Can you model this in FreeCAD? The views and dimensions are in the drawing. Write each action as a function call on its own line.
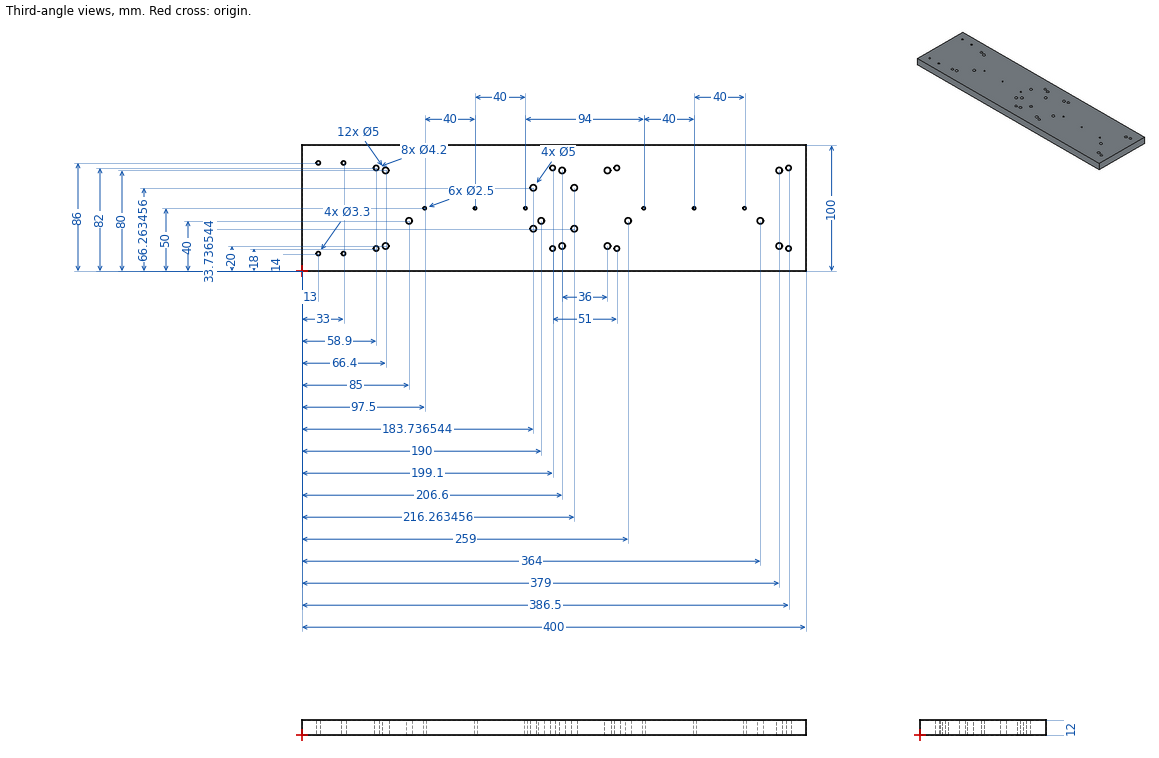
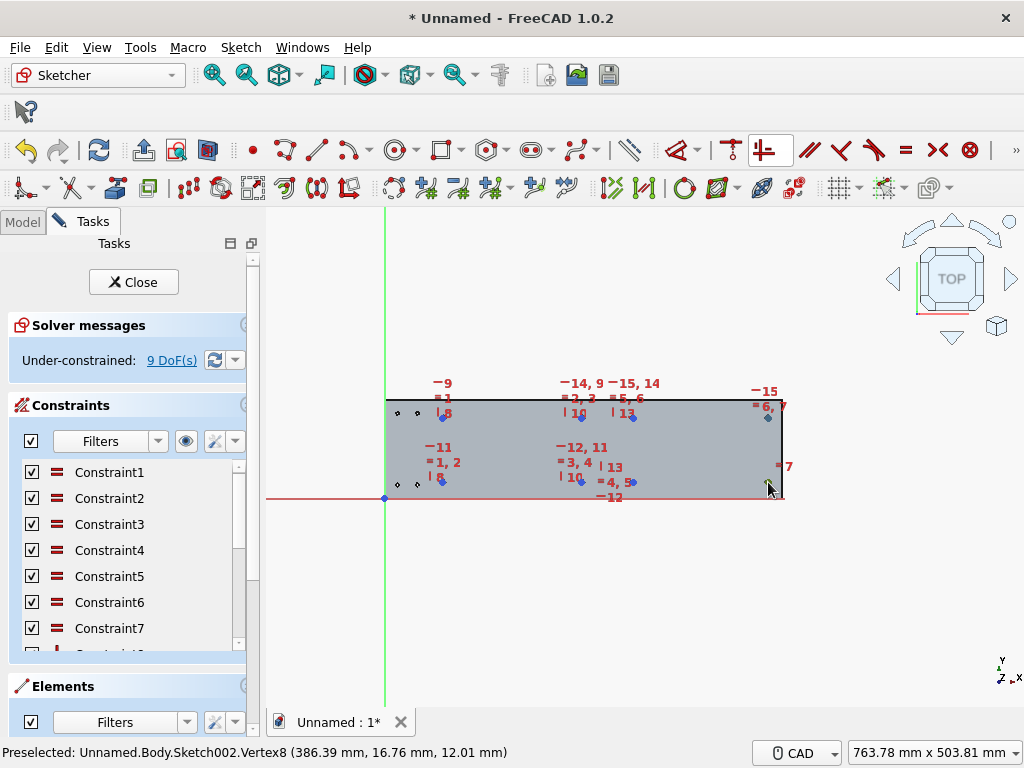
click(788, 150)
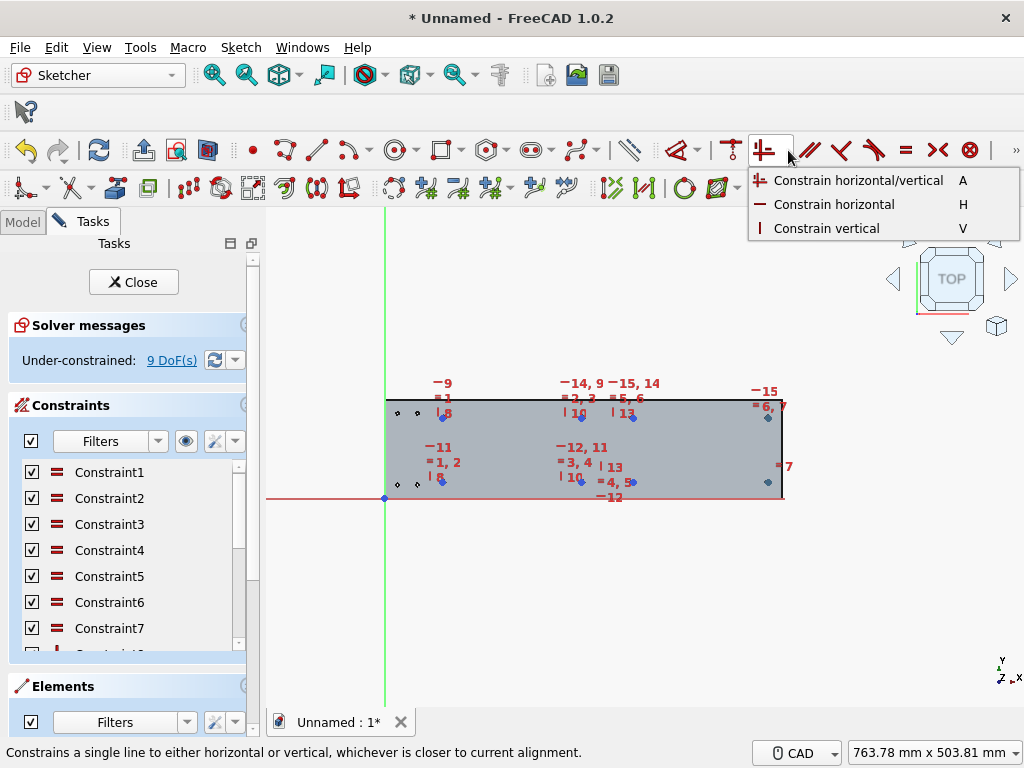
click(884, 228)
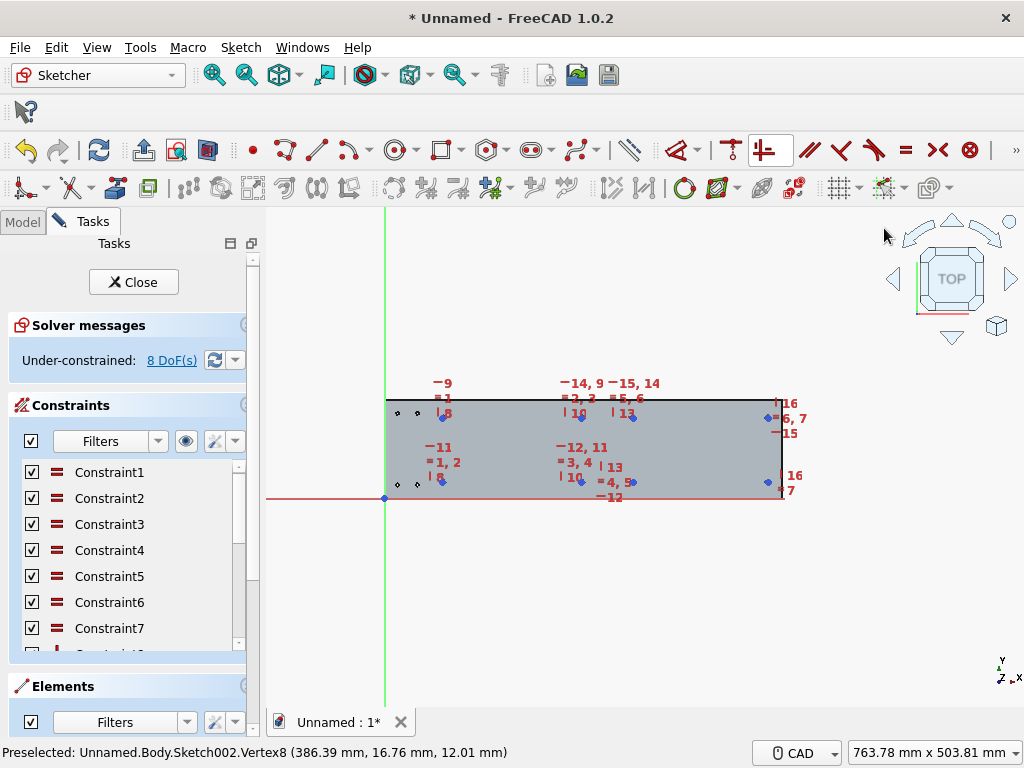
click(633, 482)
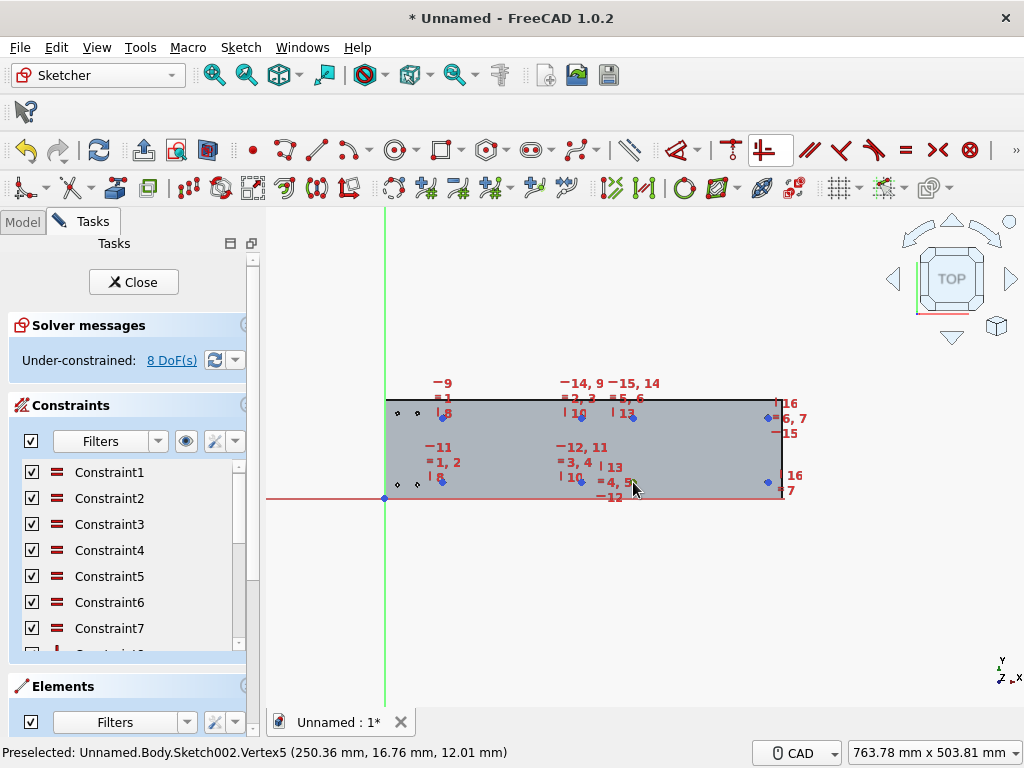
click(768, 482)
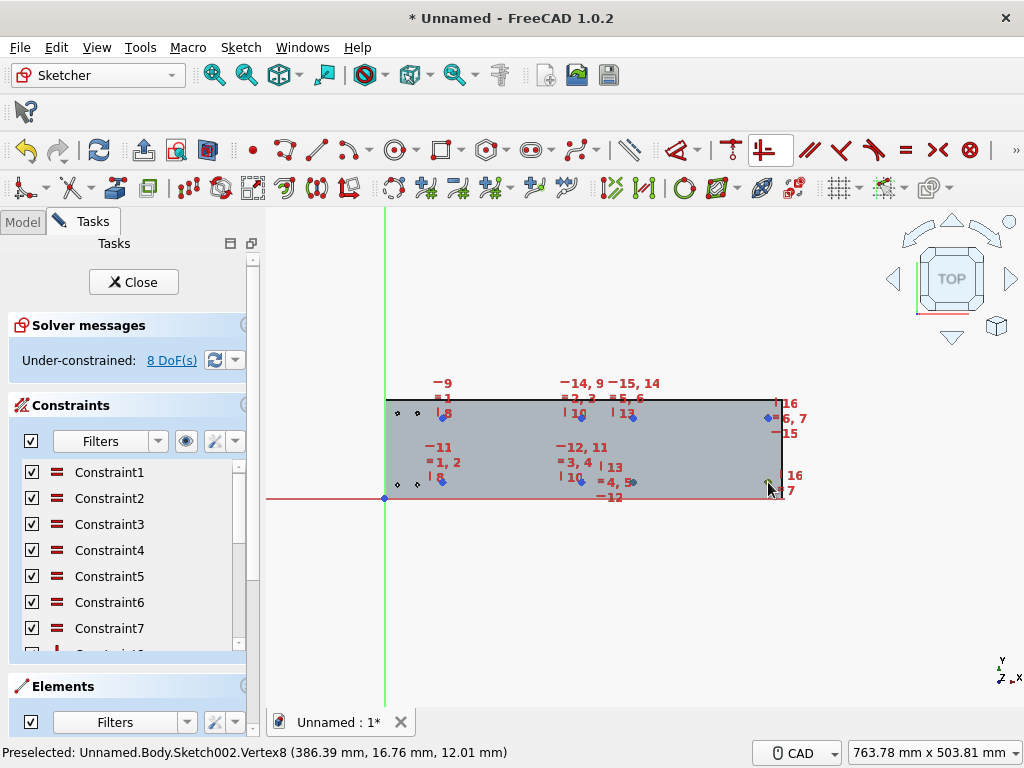
click(788, 150)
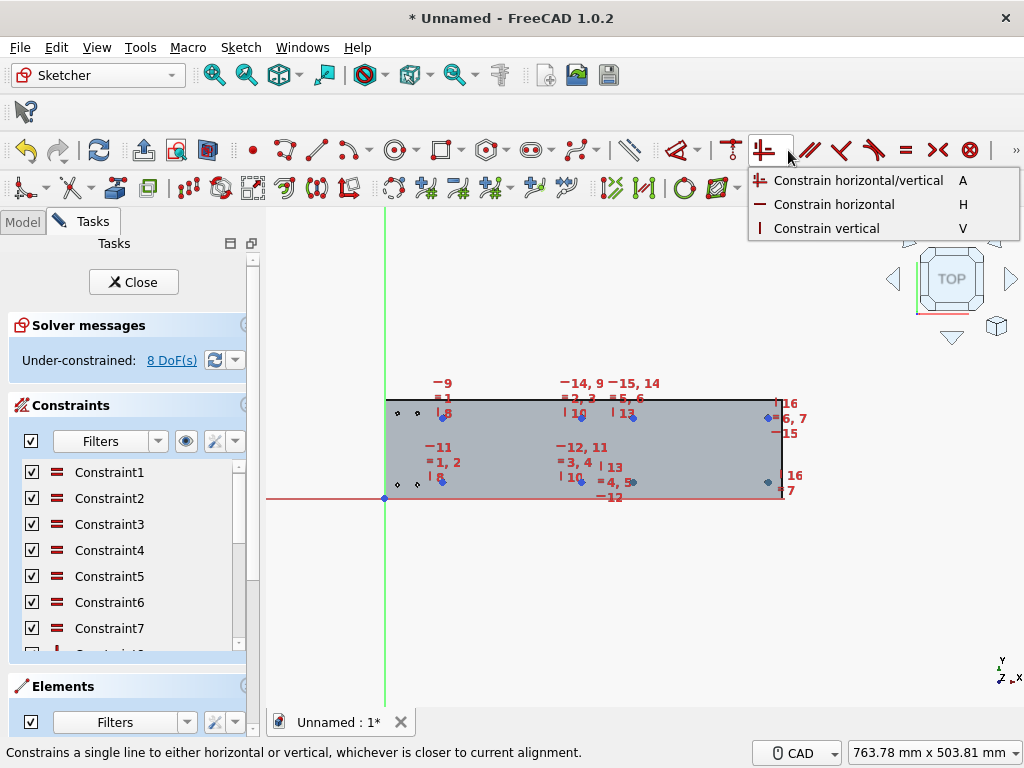
click(884, 204)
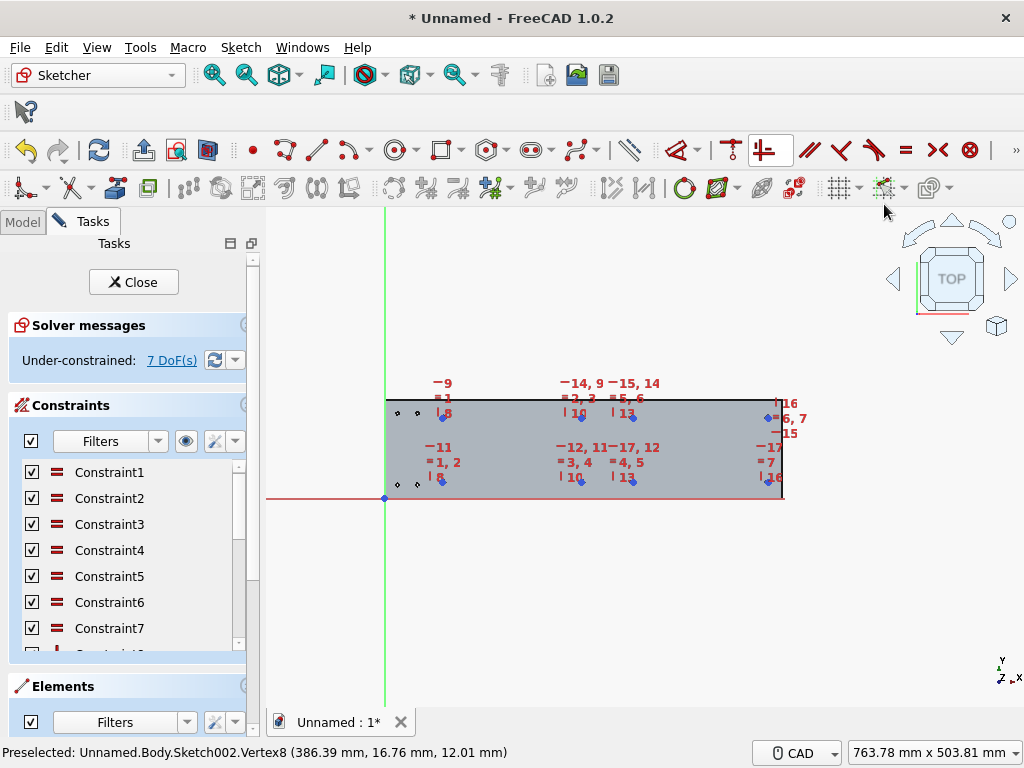
click(676, 150)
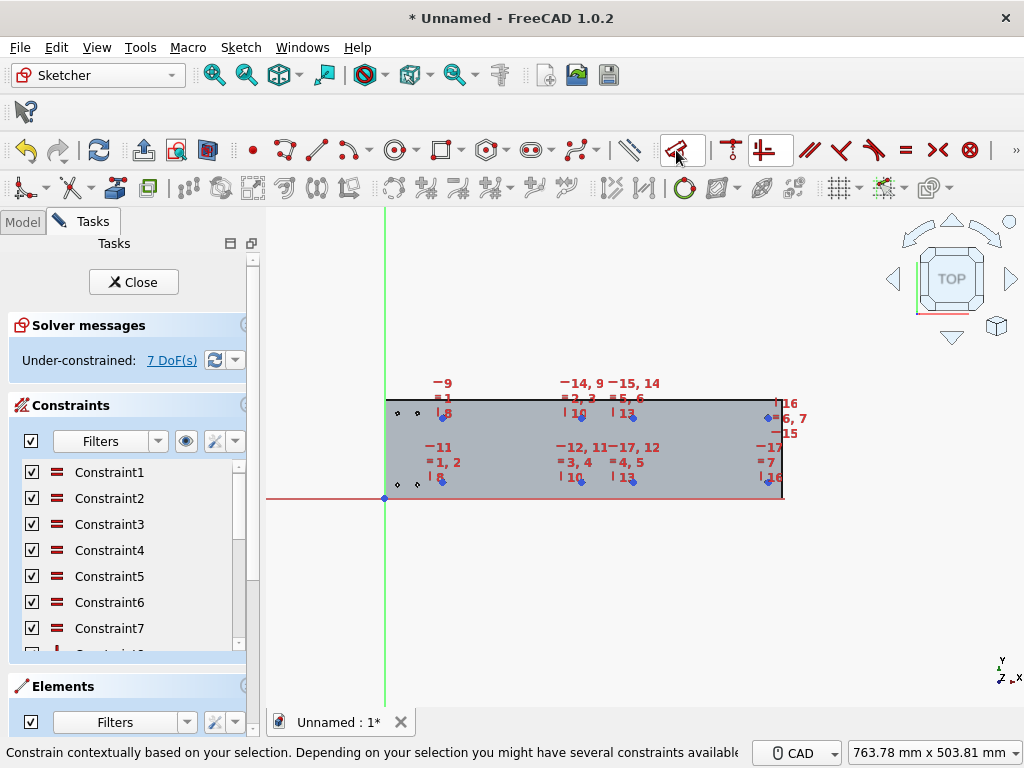
scroll(441, 416, up, 12)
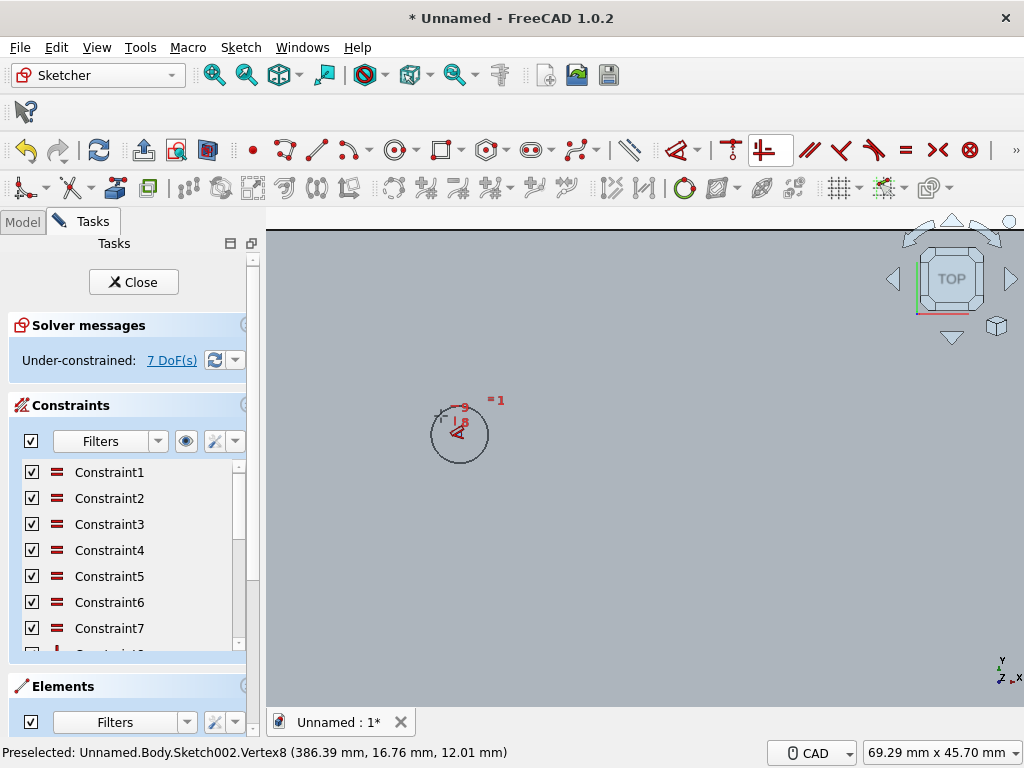
click(440, 415)
click(417, 392)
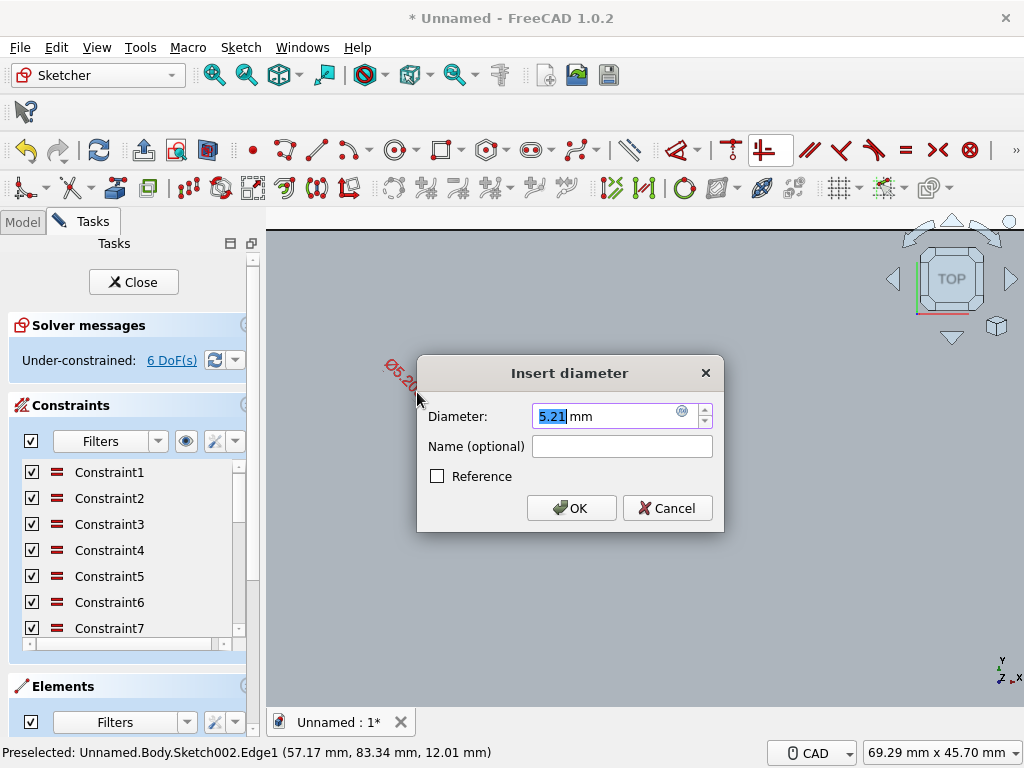
text(4.2)
key(Return)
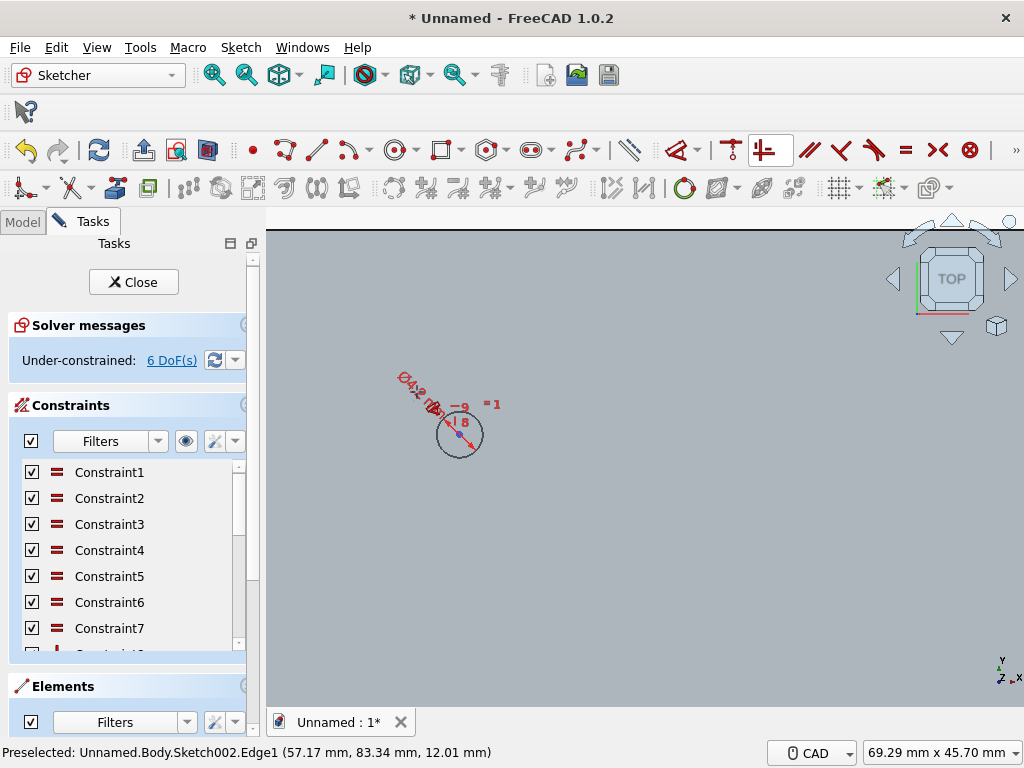
scroll(440, 416, down, 12)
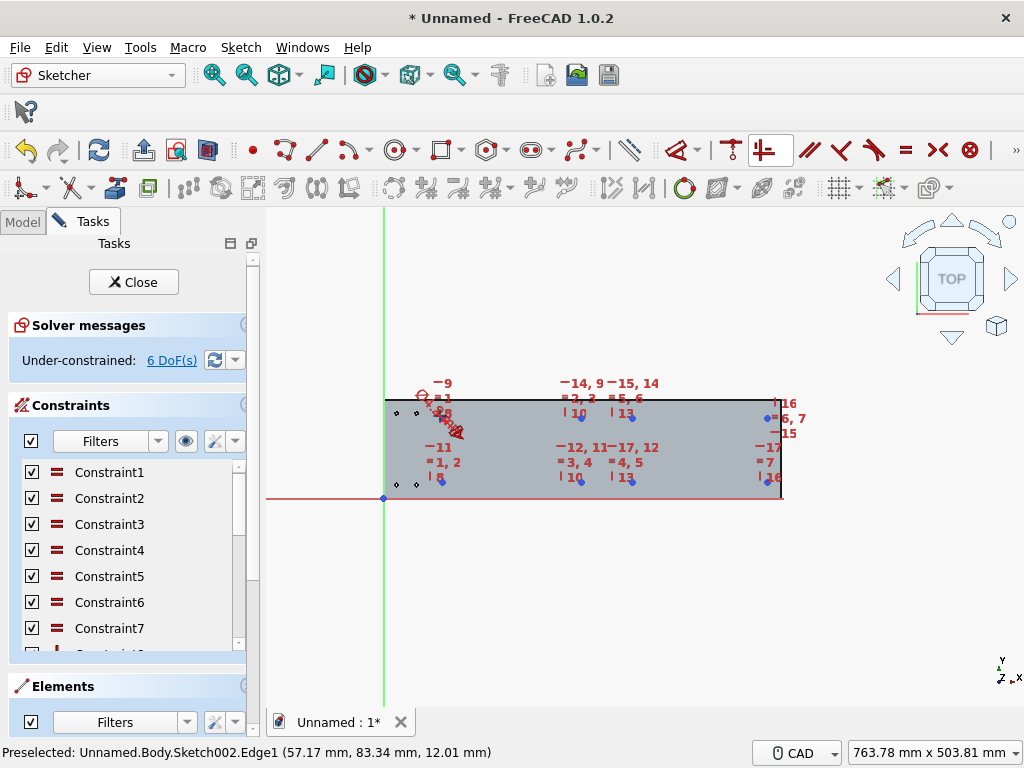
click(442, 418)
click(350, 458)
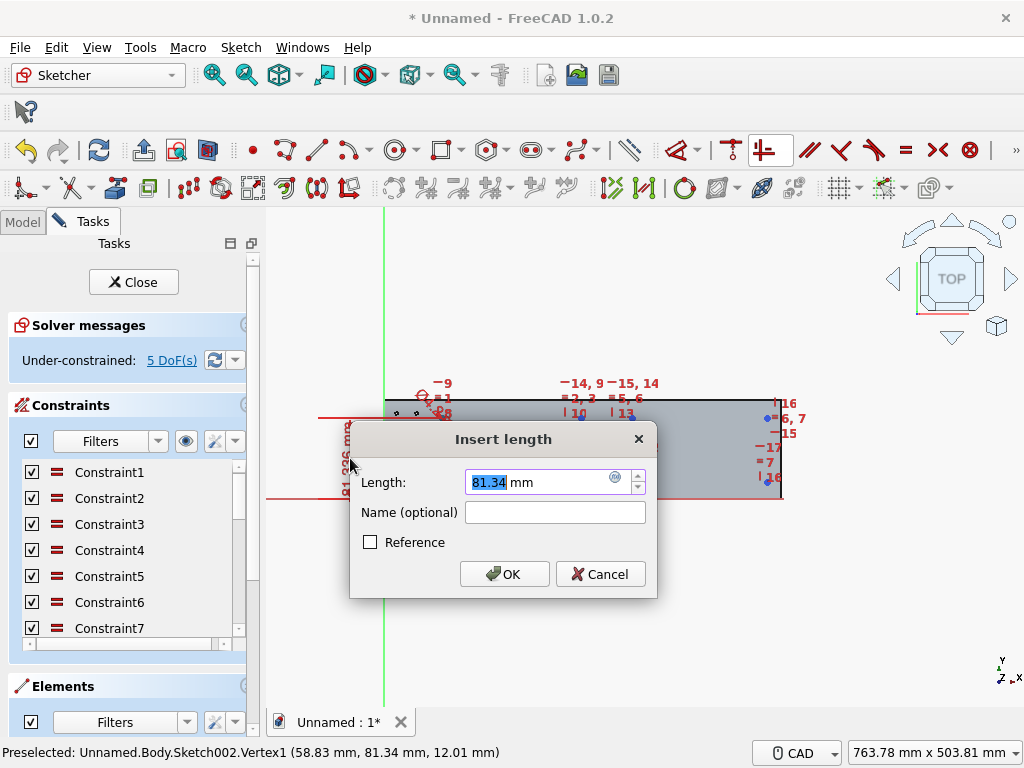
text(82)
key(Return)